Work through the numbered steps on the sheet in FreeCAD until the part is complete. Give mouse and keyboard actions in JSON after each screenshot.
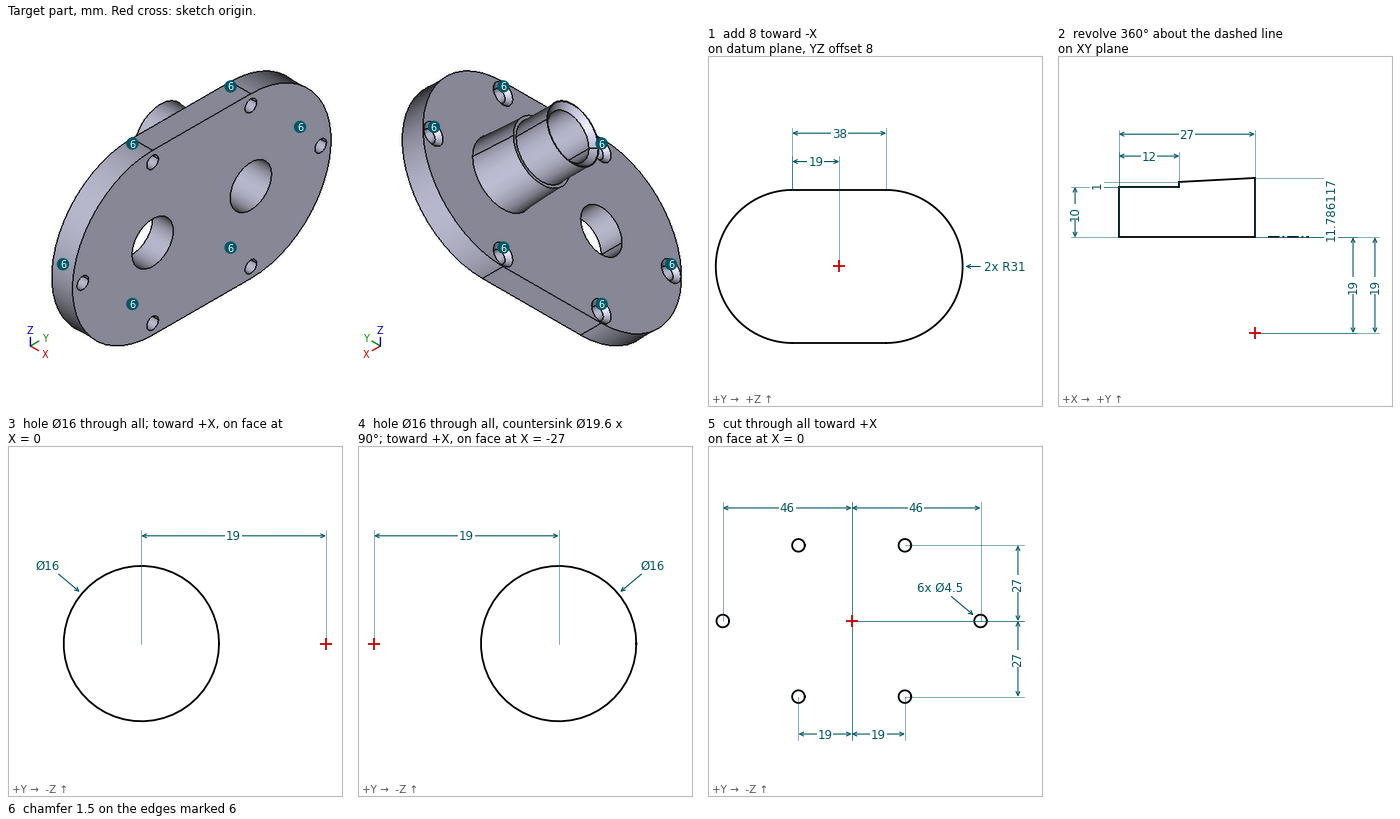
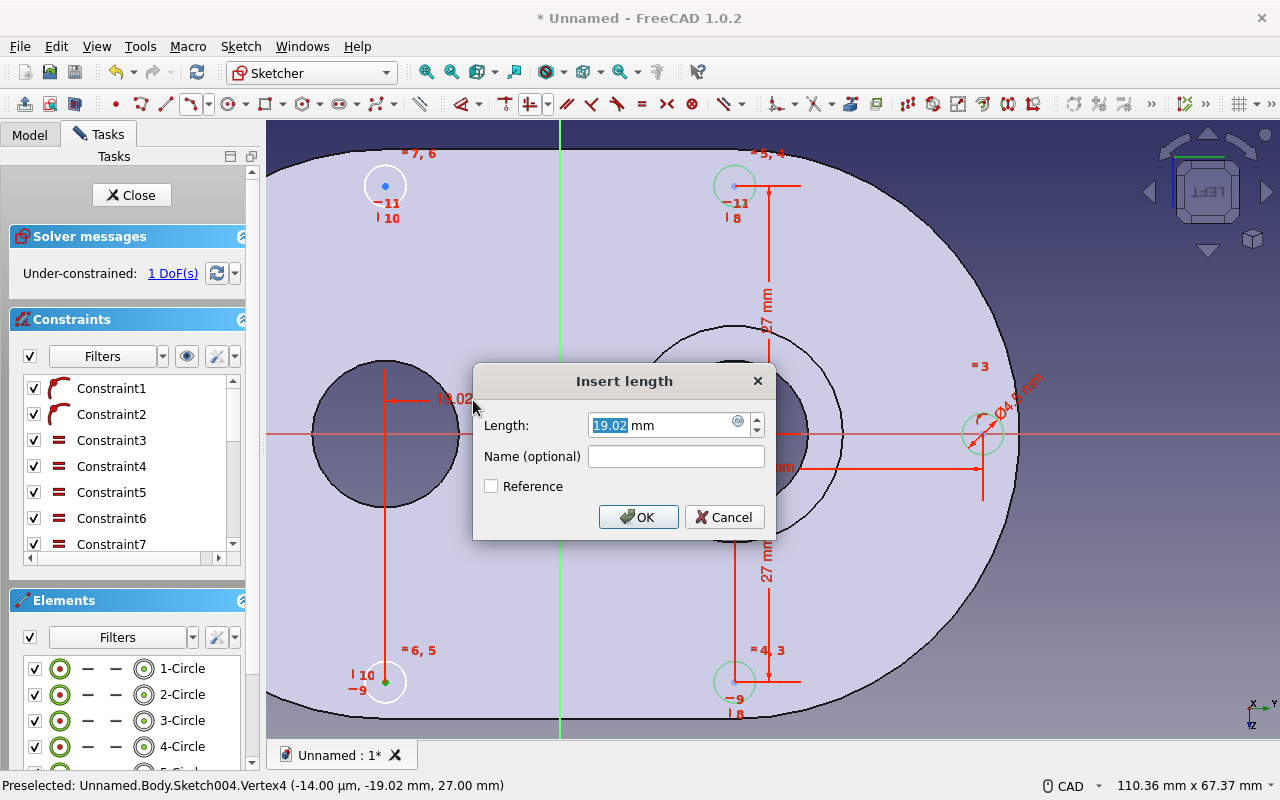
{"action": "type", "text": "19"}
{"action": "key", "text": "Return"}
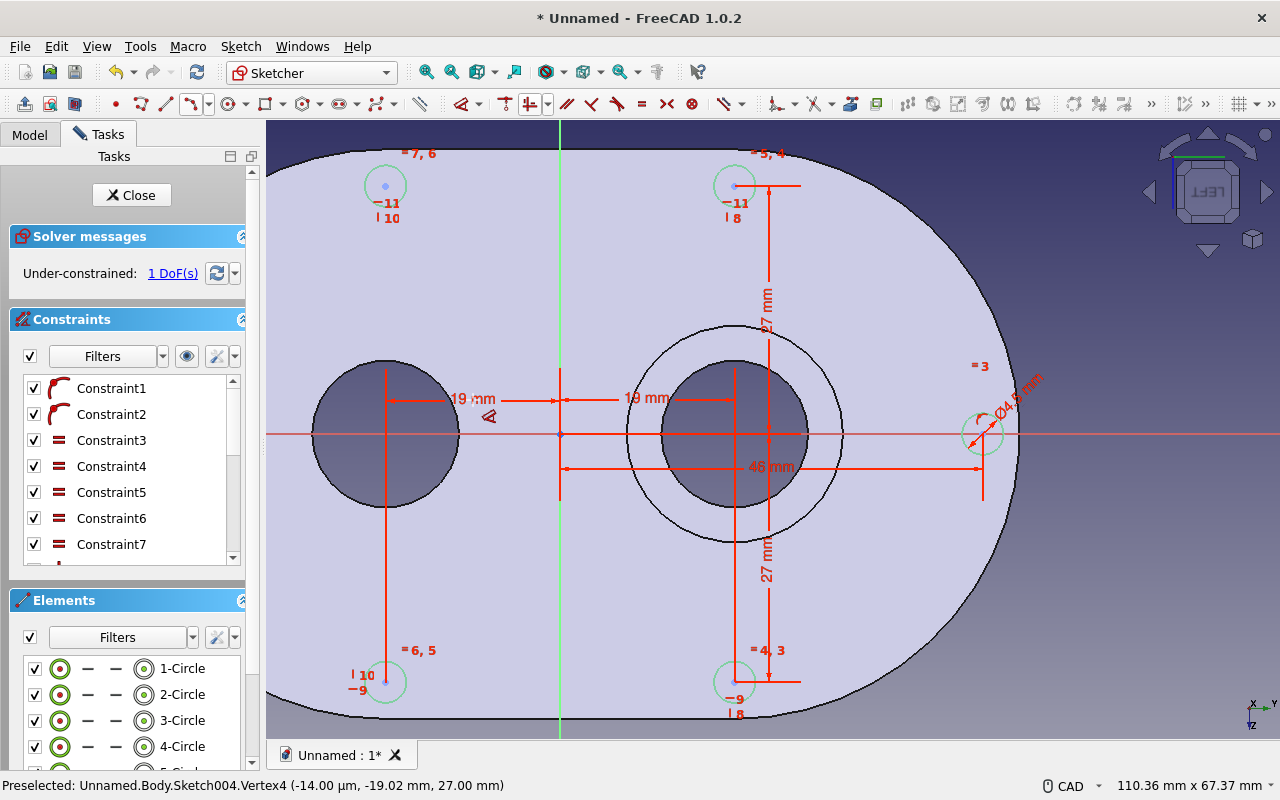
{"action": "scroll", "coordinate": [998, 420], "scroll_direction": "down", "scroll_amount": 2}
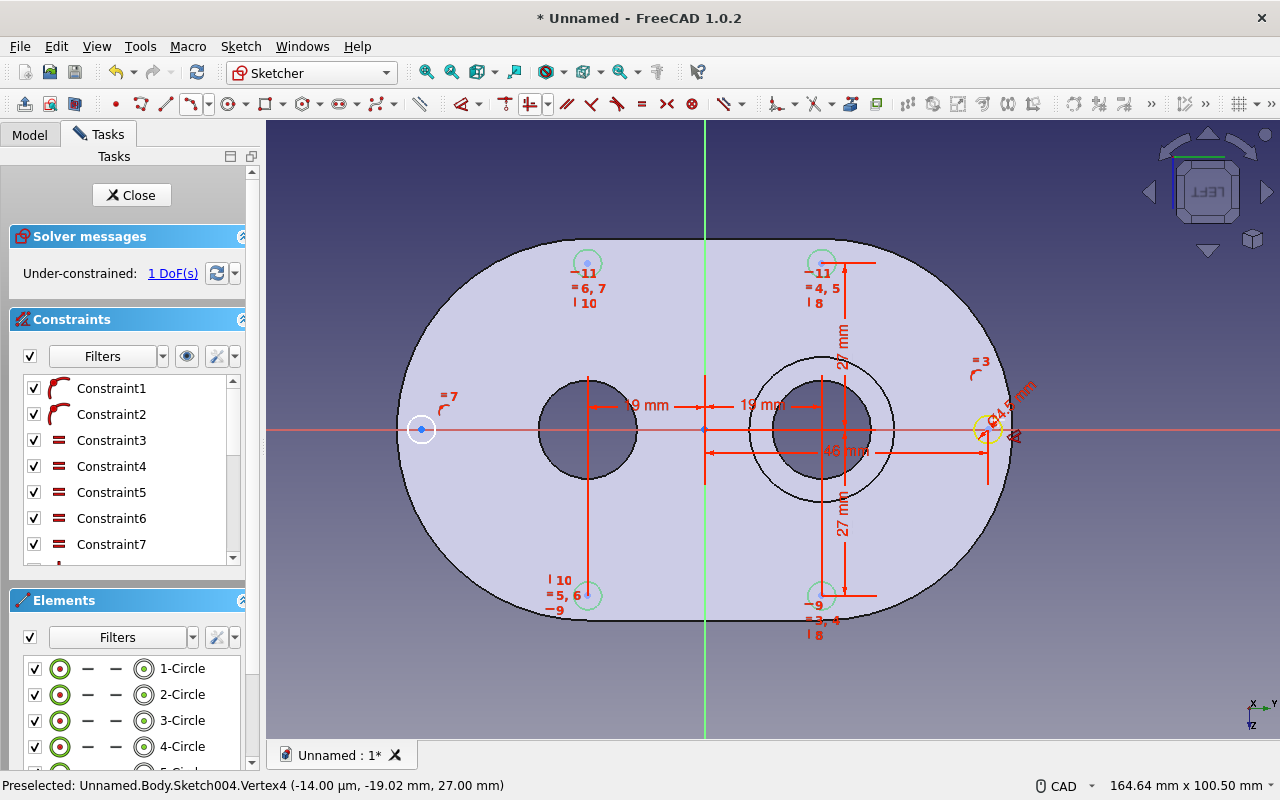
{"action": "left_click", "coordinate": [422, 430]}
{"action": "left_click", "coordinate": [563, 464]}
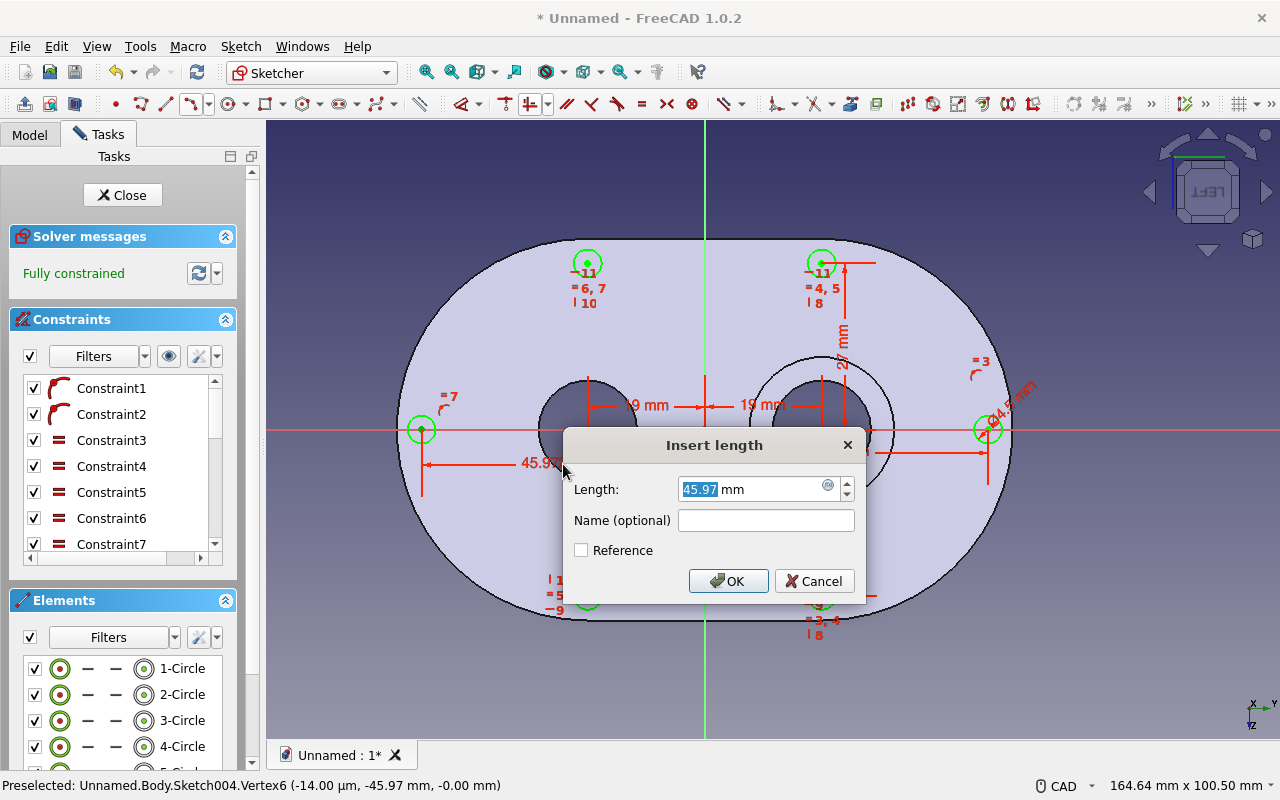
{"action": "type", "text": "46"}
{"action": "key", "text": "Return"}
{"action": "key", "text": "Escape"}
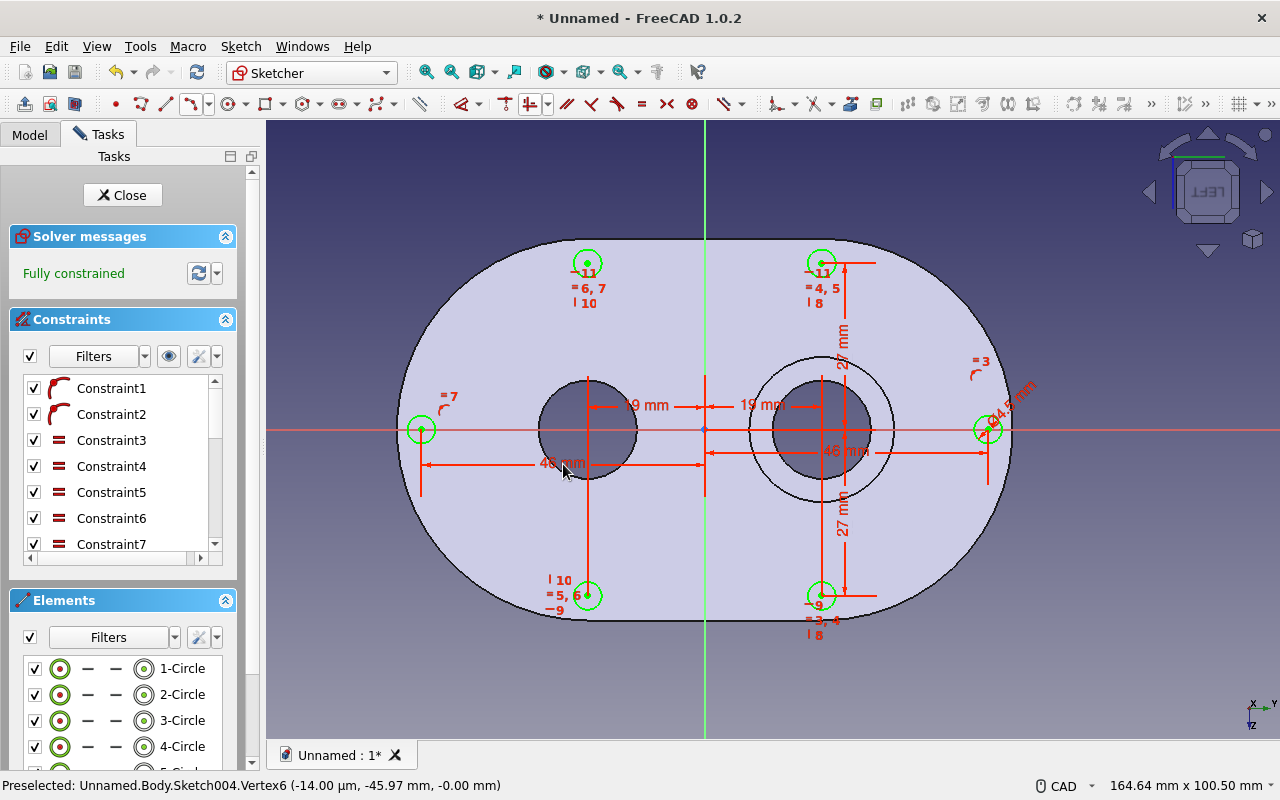
{"action": "left_click", "coordinate": [123, 195]}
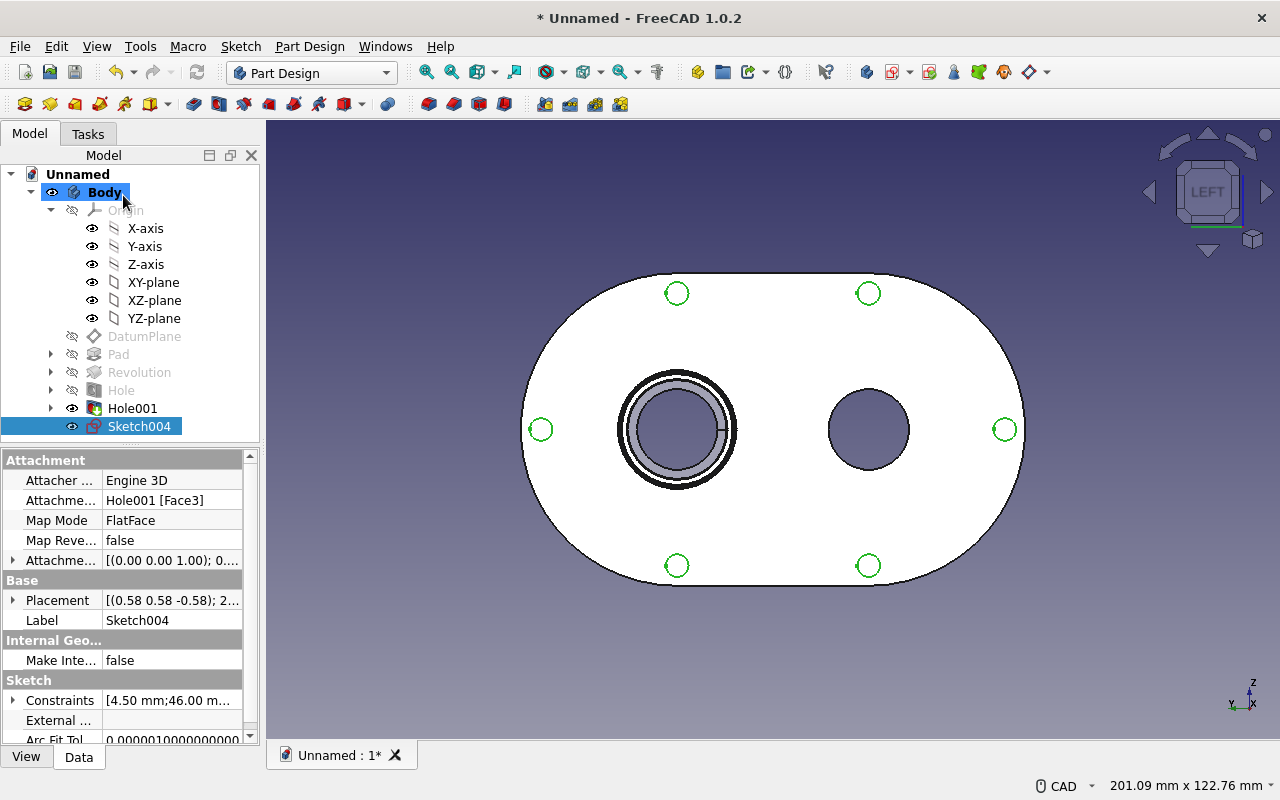
{"action": "left_click", "coordinate": [194, 104]}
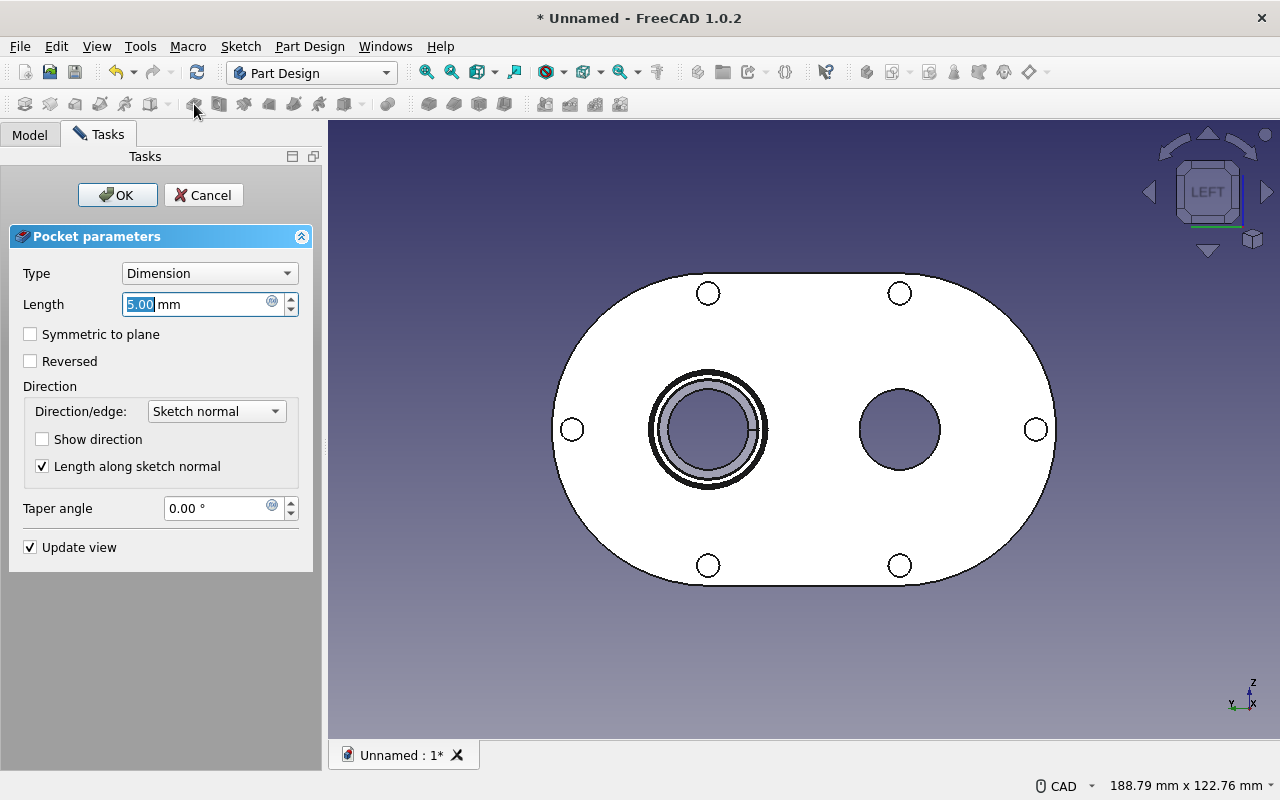
{"action": "left_click", "coordinate": [210, 274]}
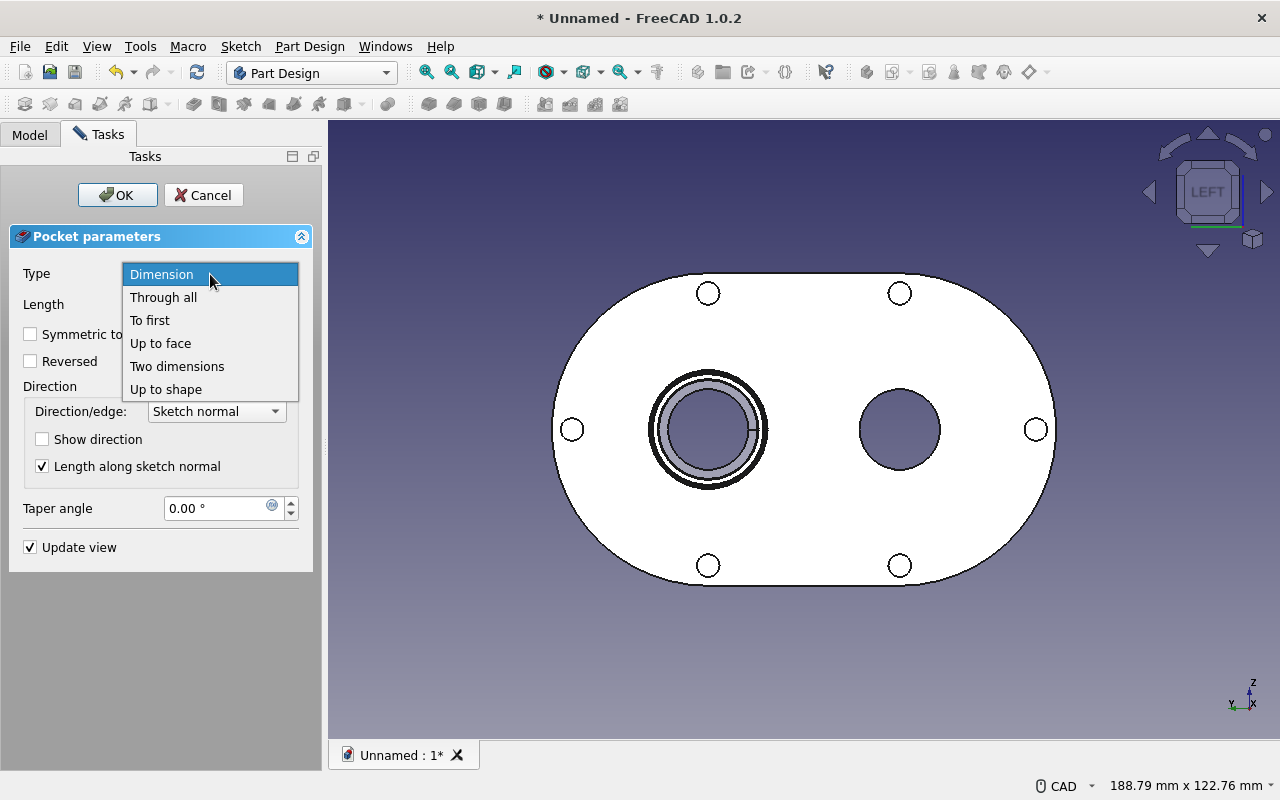
{"action": "left_click", "coordinate": [208, 298]}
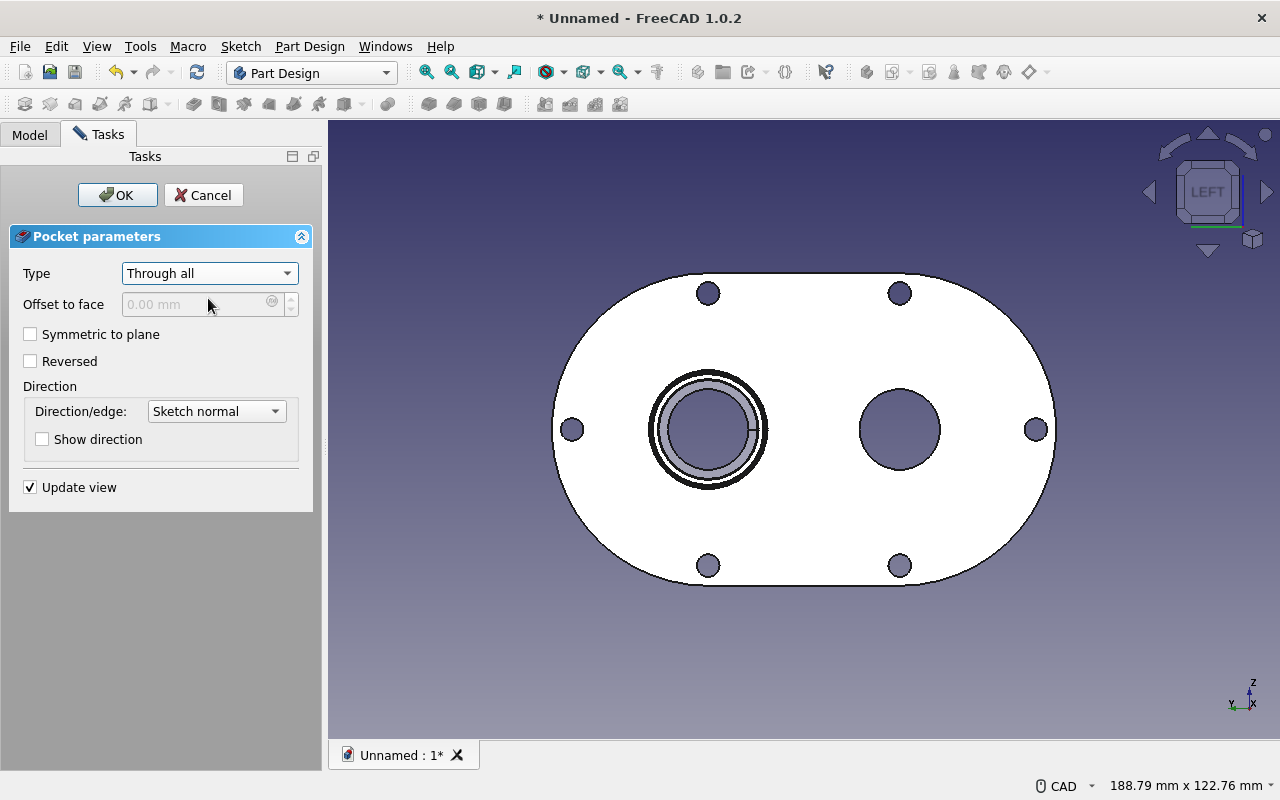
{"action": "left_click", "coordinate": [118, 195]}